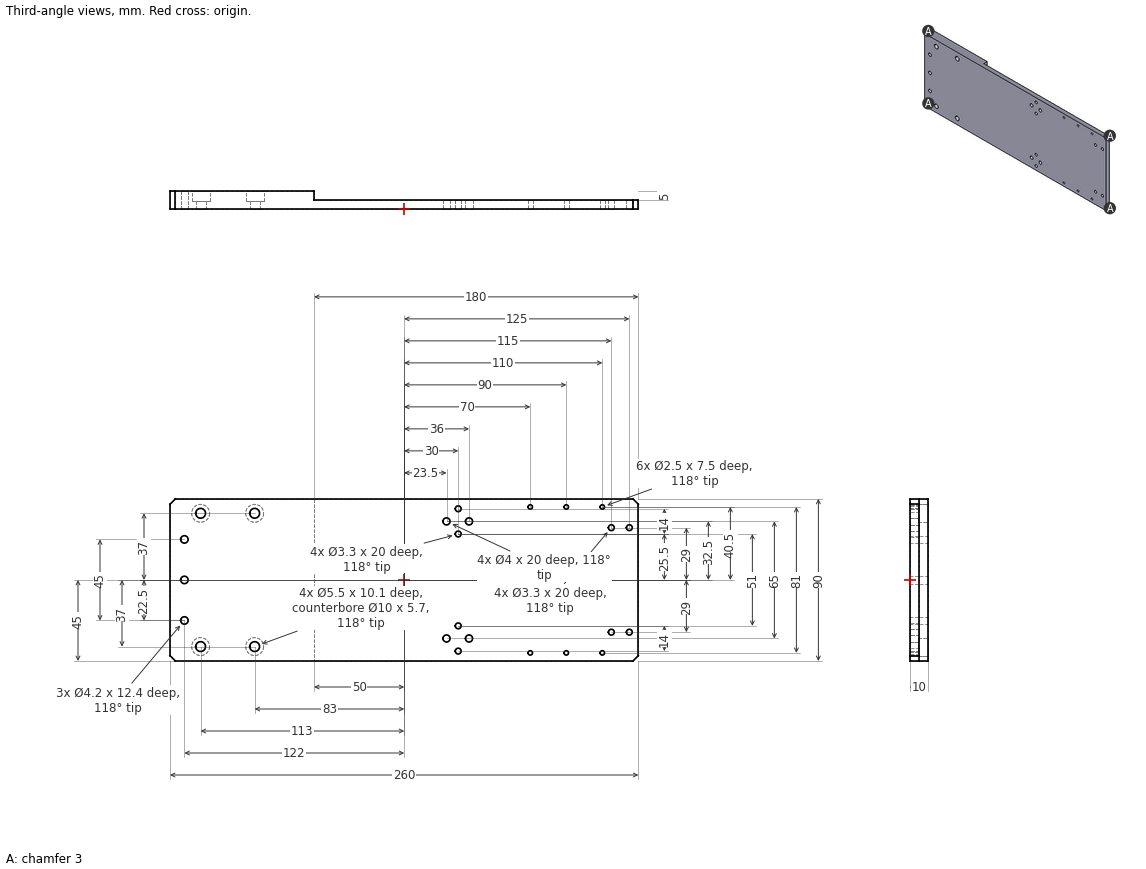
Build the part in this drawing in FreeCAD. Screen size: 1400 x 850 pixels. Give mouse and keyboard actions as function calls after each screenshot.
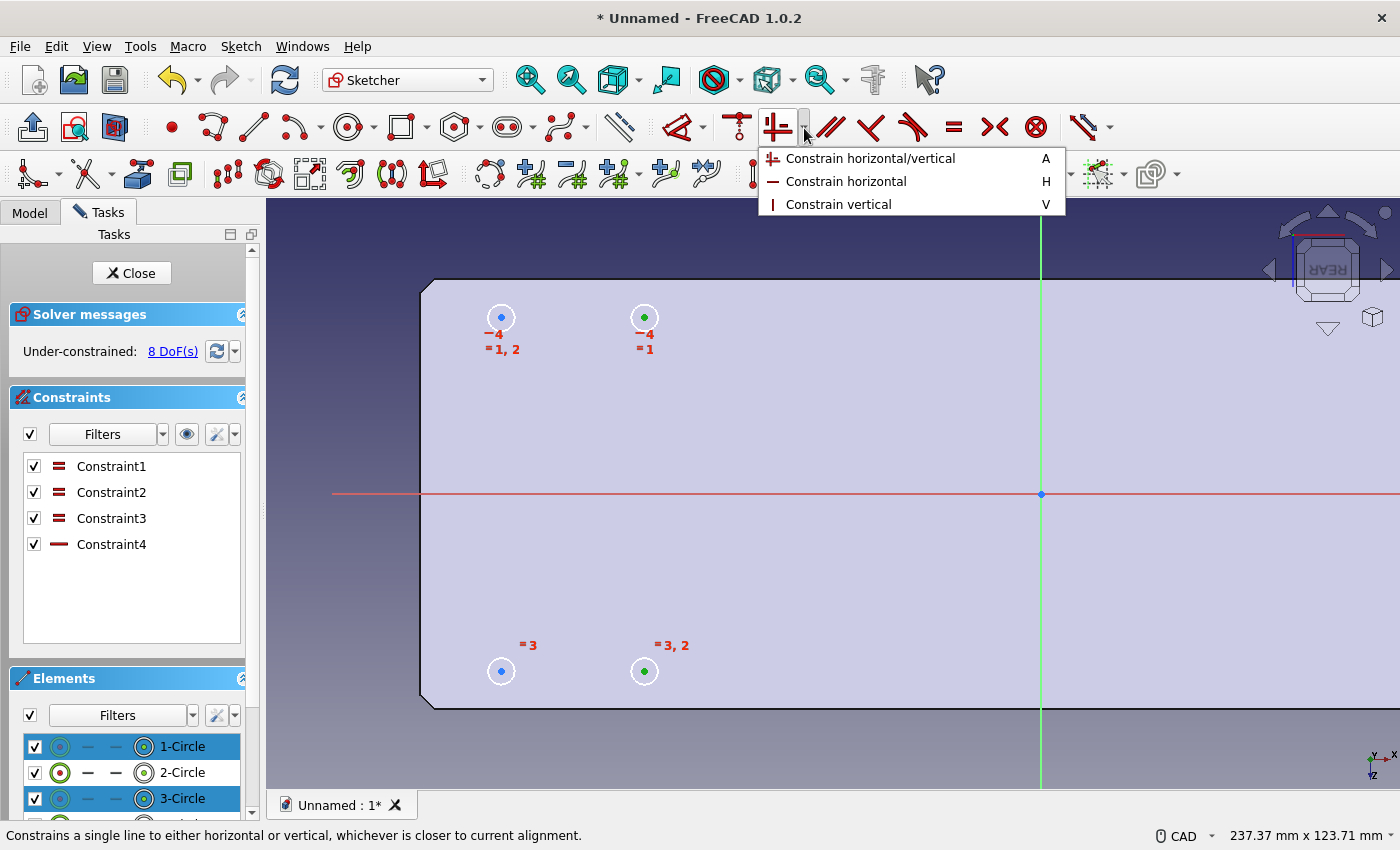
click(912, 204)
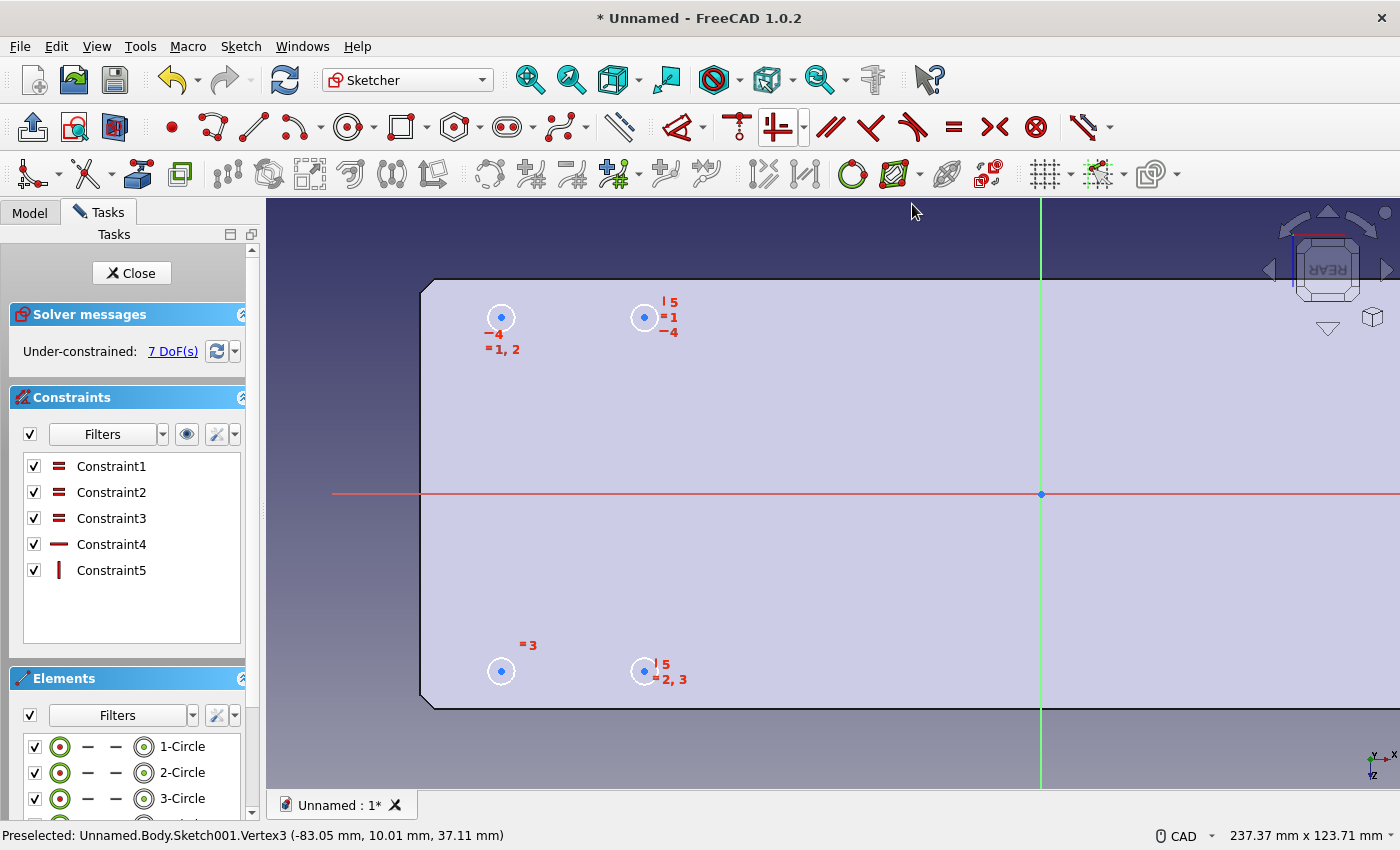
click(501, 318)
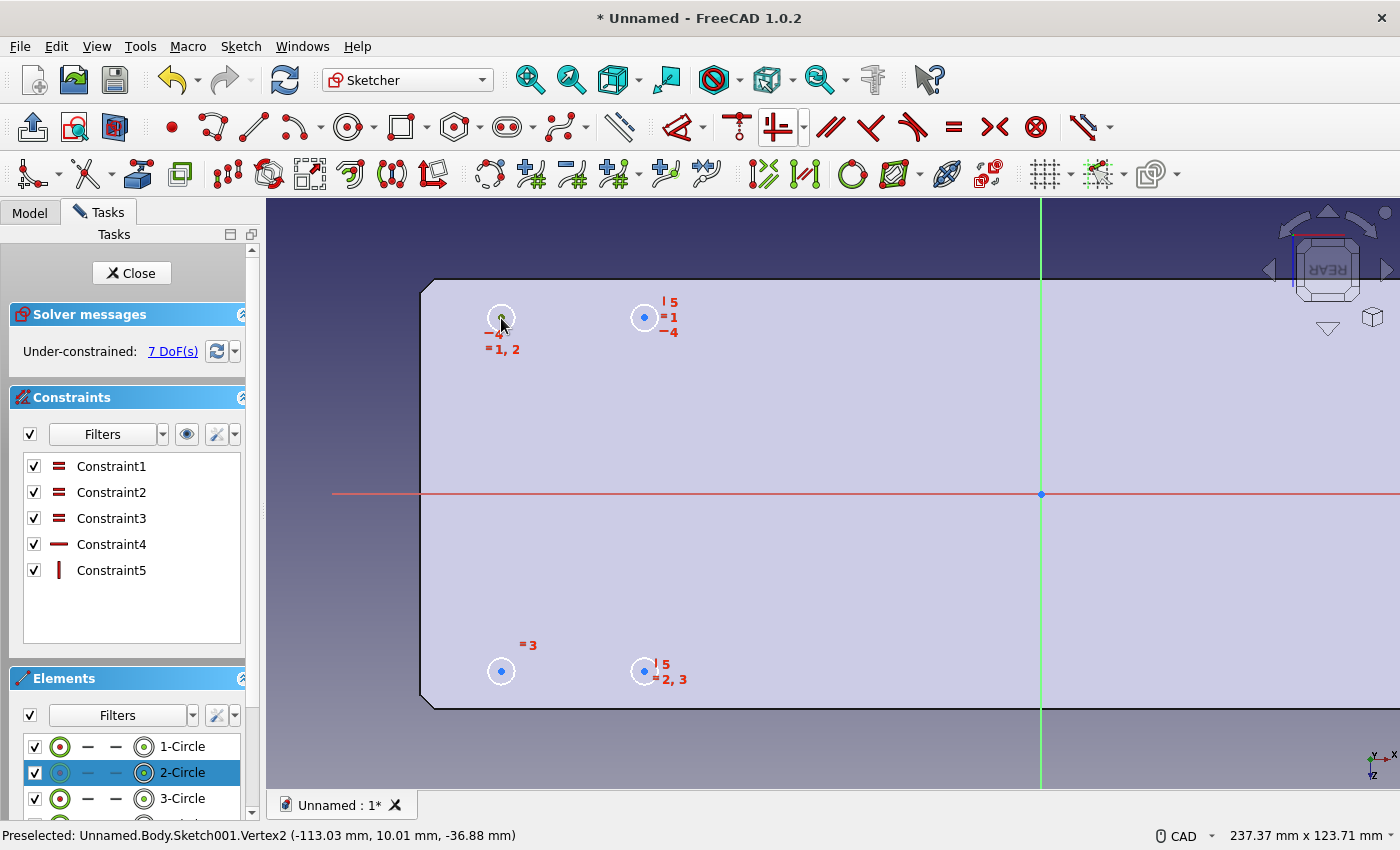
click(501, 671)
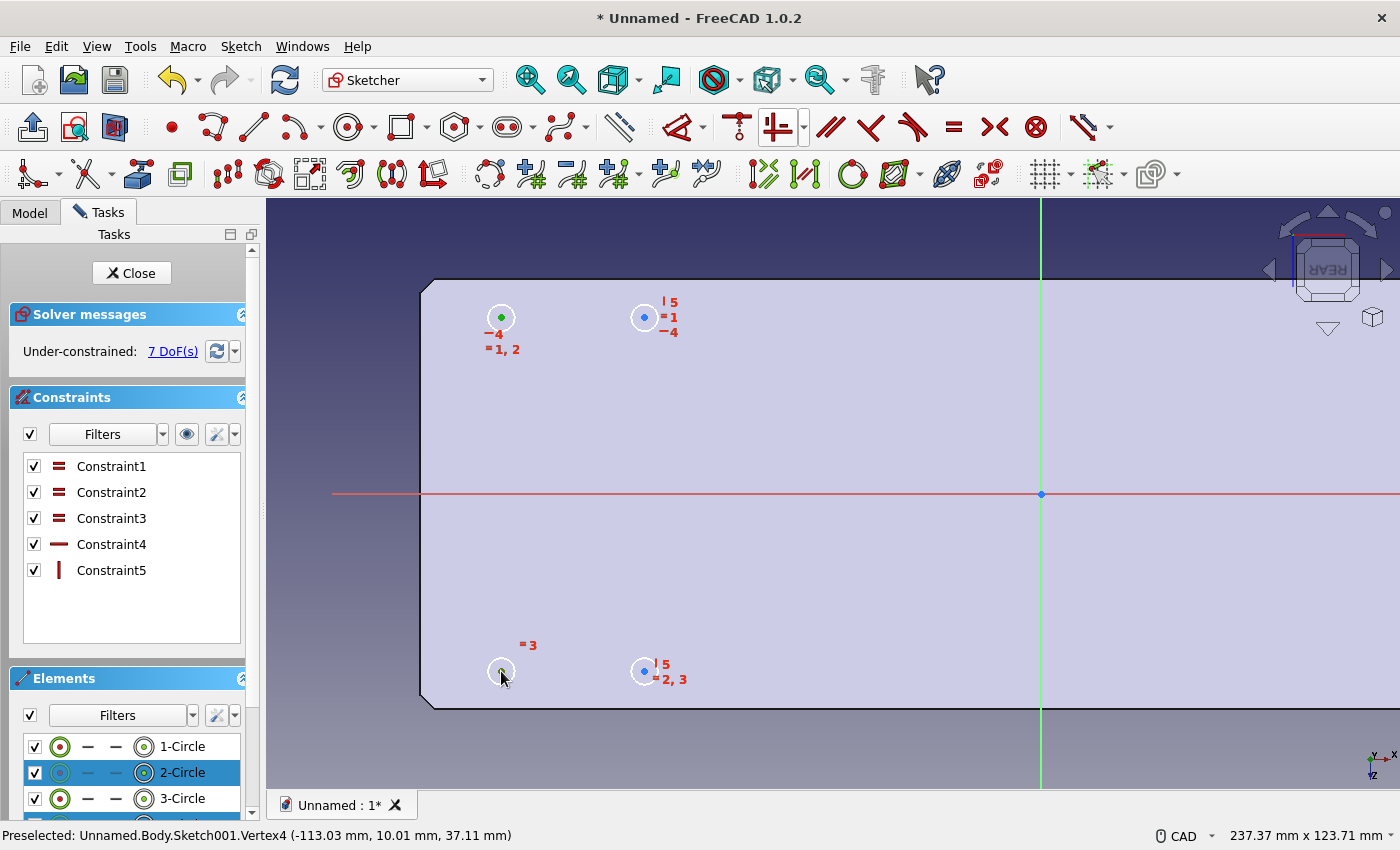
key(v)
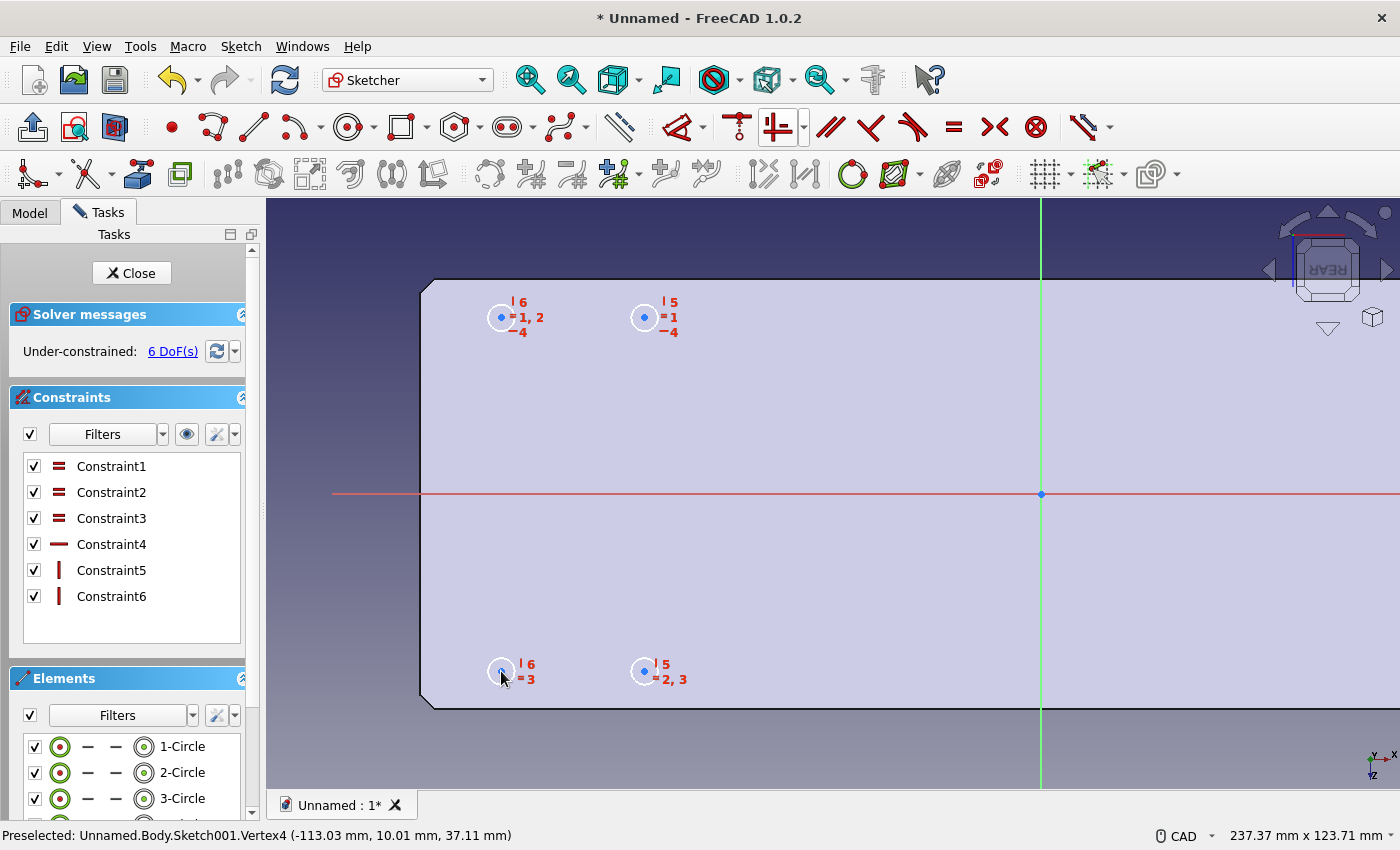
click(645, 671)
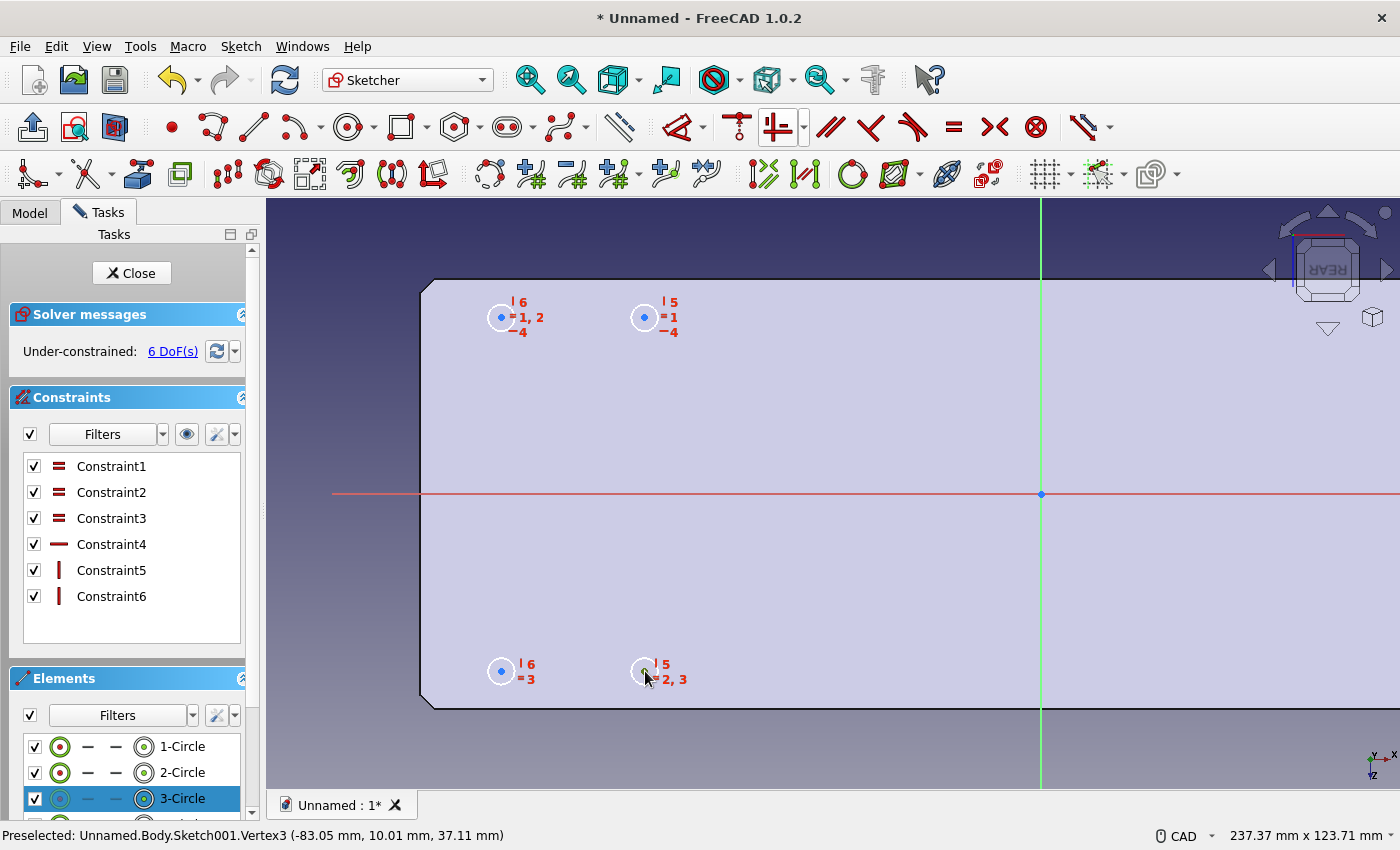
click(501, 671)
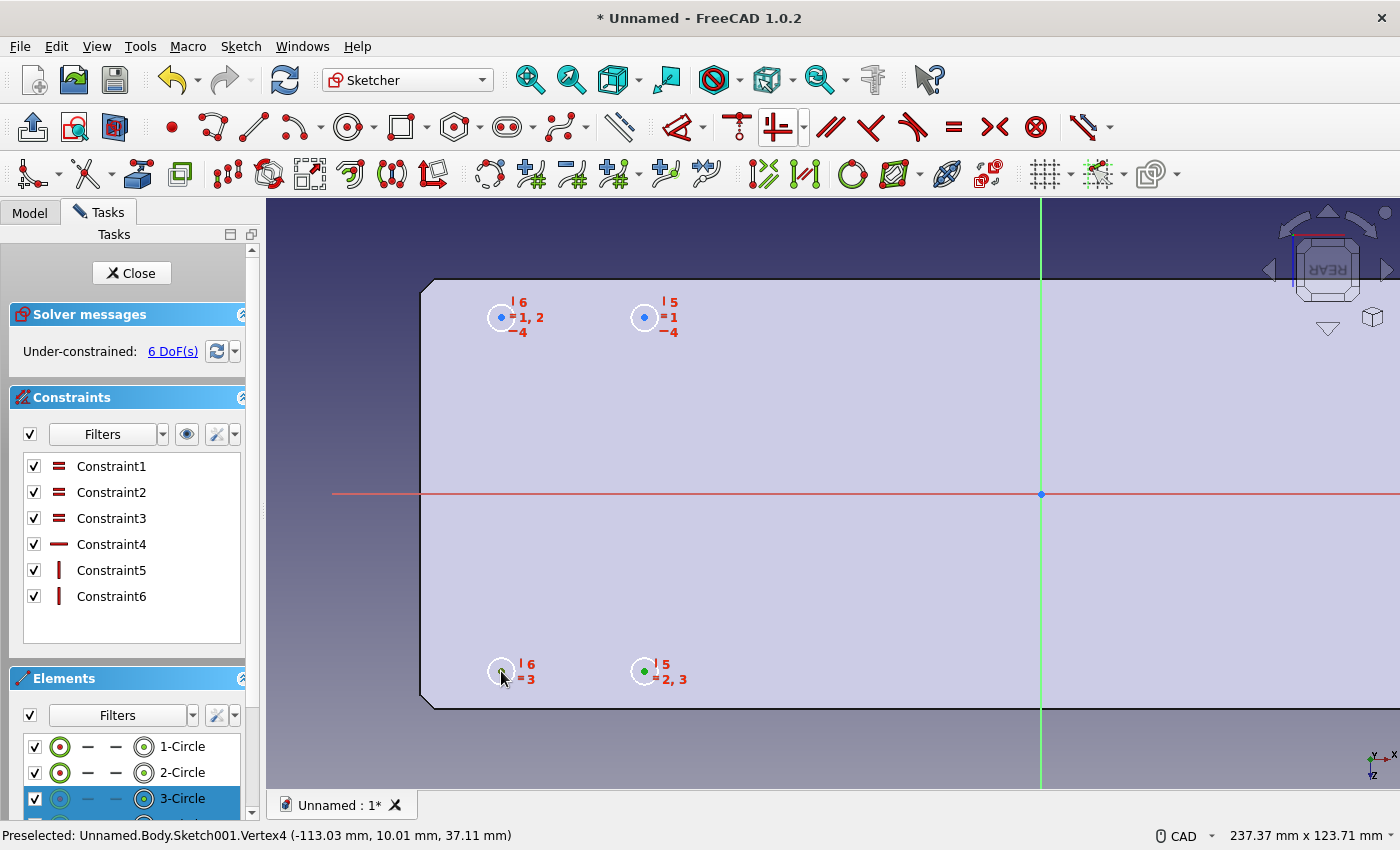
click(804, 128)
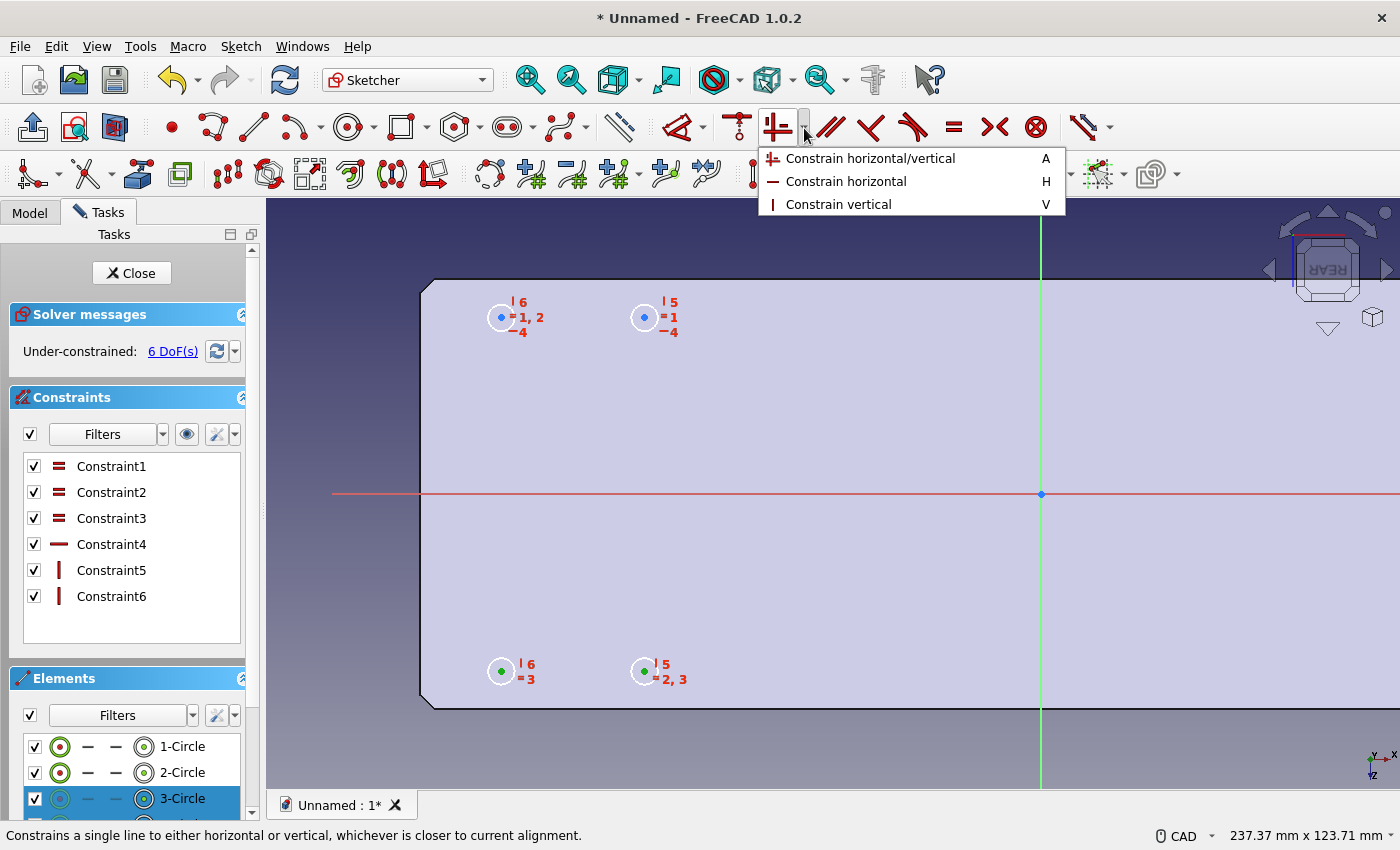
click(912, 182)